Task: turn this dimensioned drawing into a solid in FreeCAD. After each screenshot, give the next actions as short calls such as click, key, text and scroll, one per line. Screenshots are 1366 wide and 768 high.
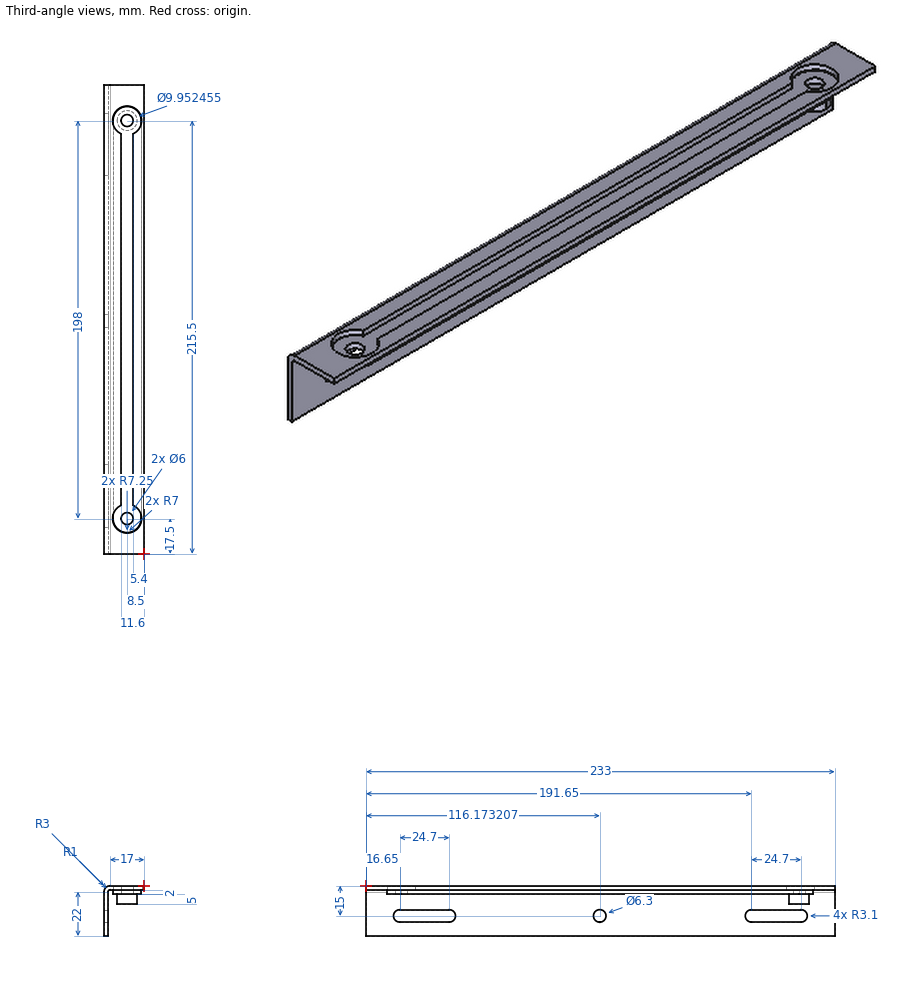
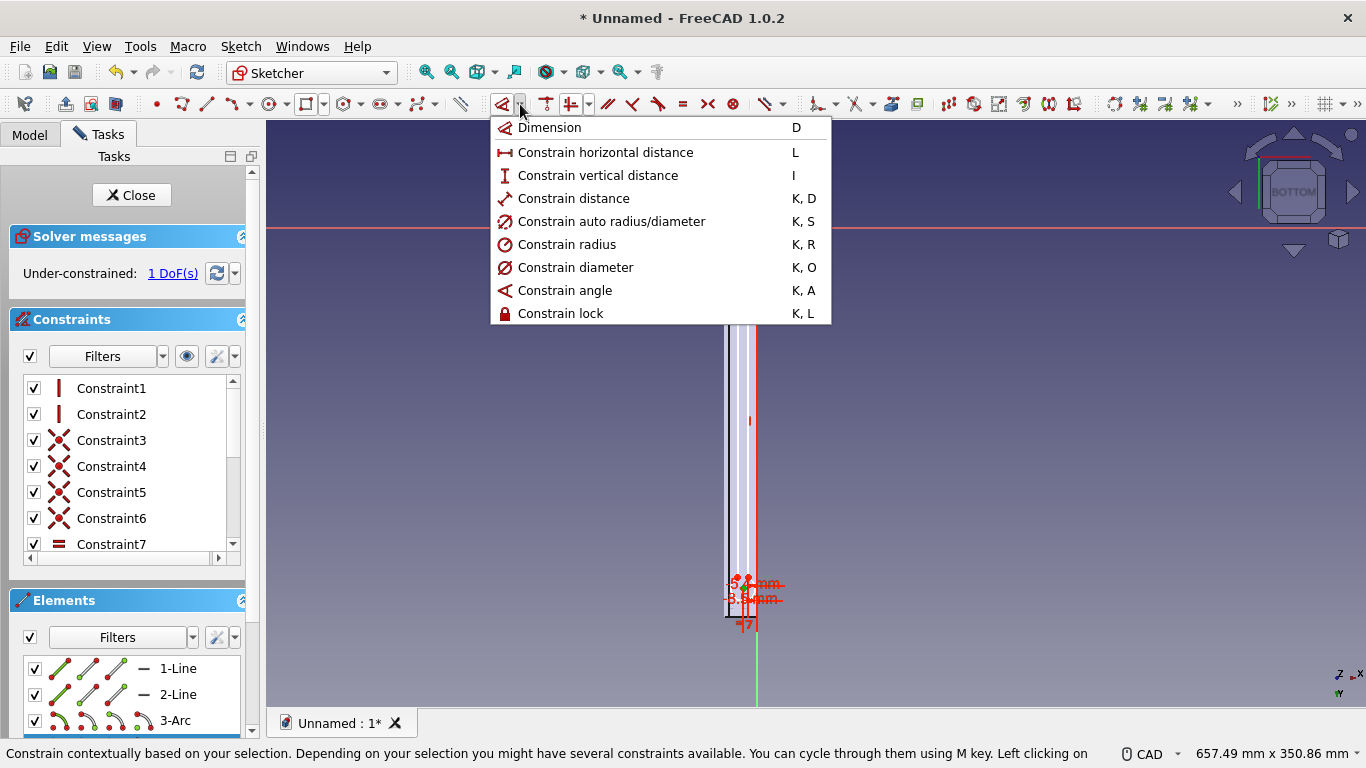
click(661, 176)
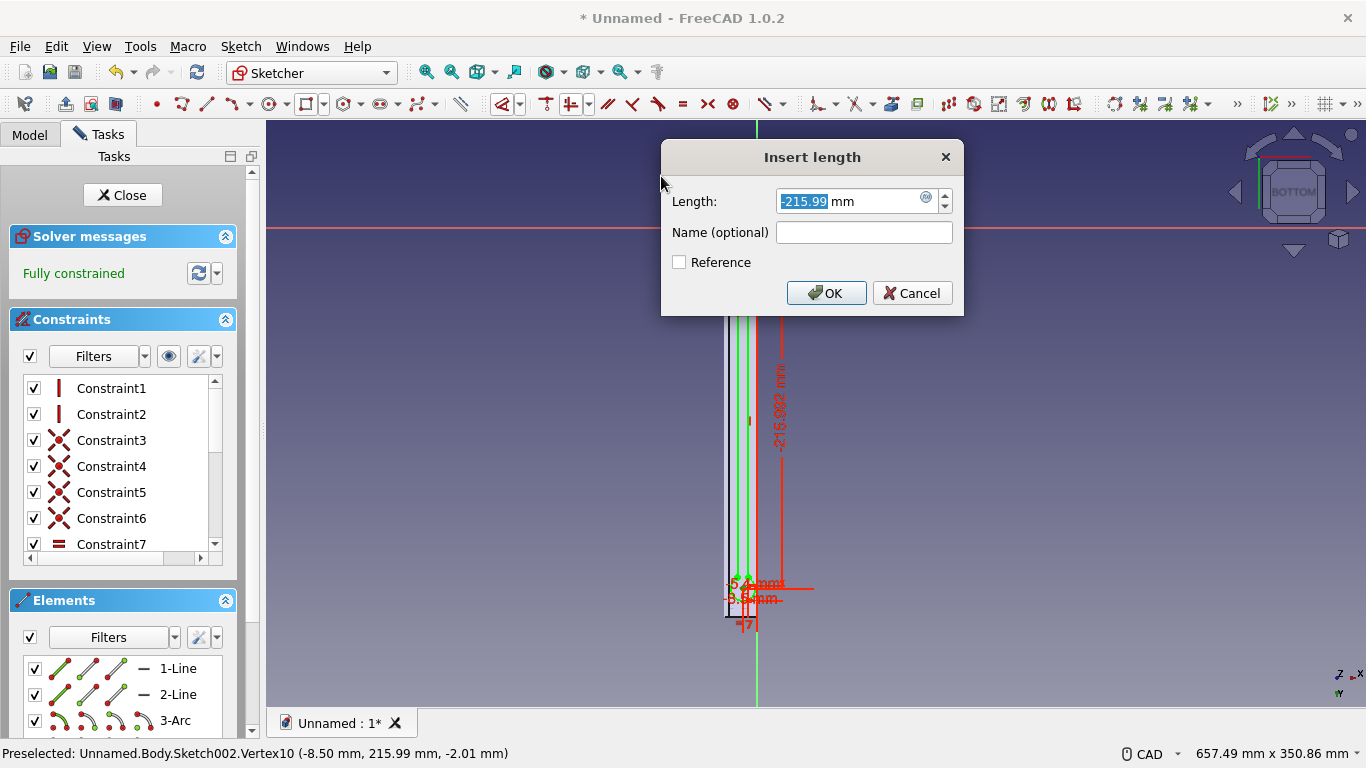
text(-215.5)
key(Return)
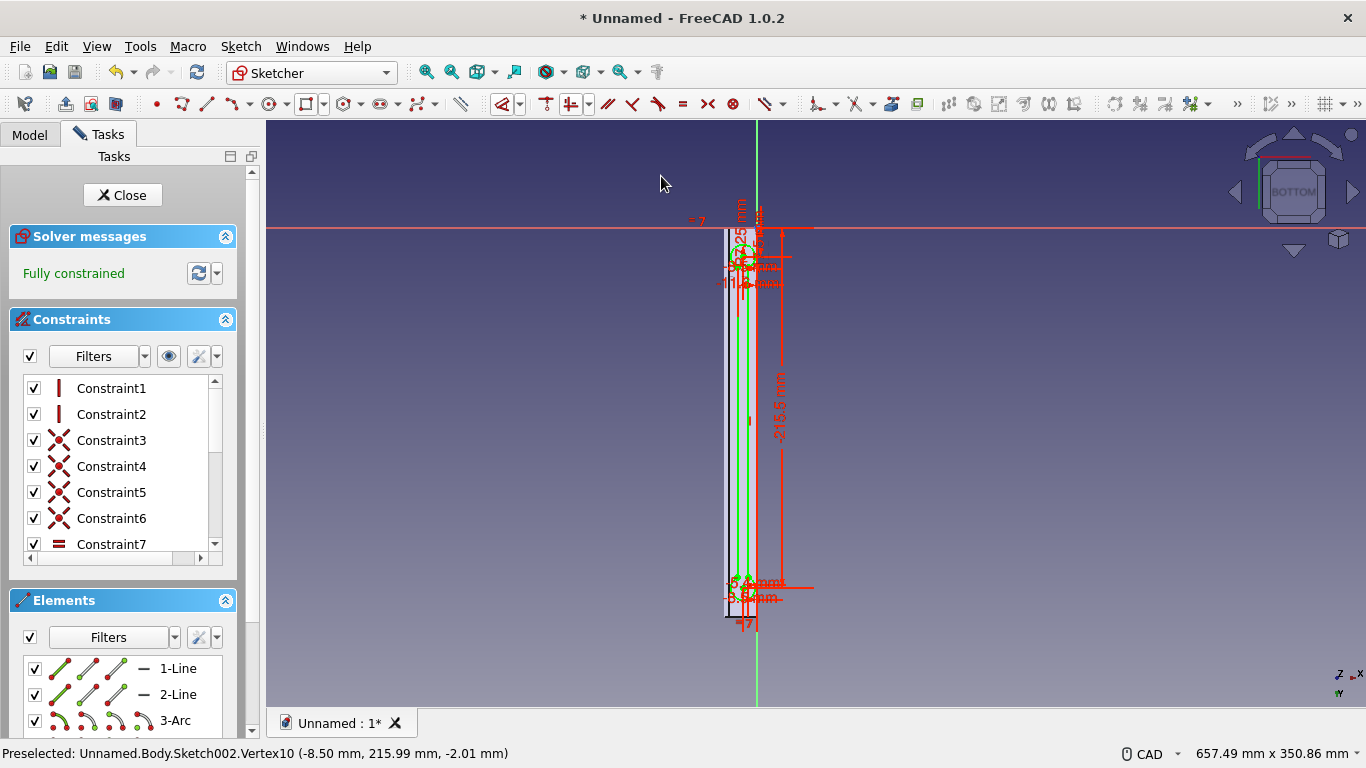
click(123, 195)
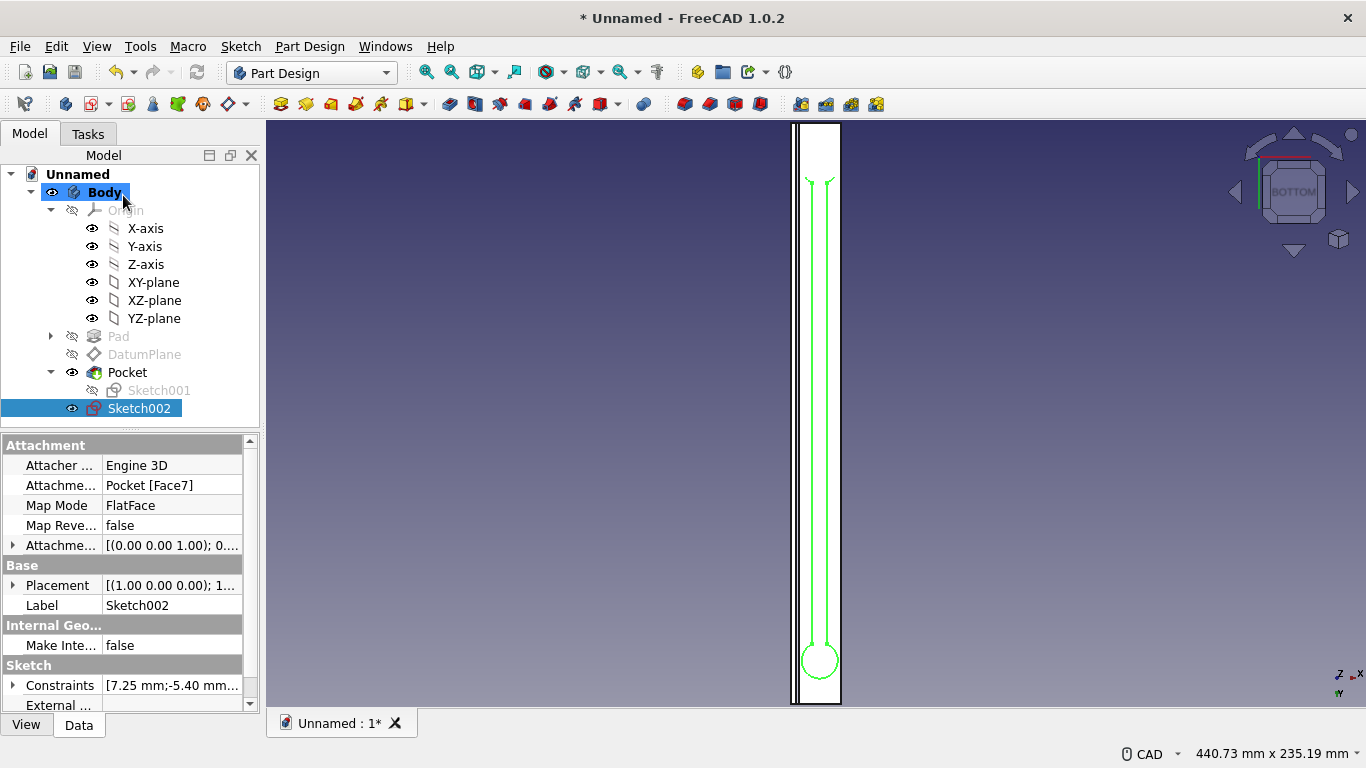
click(450, 104)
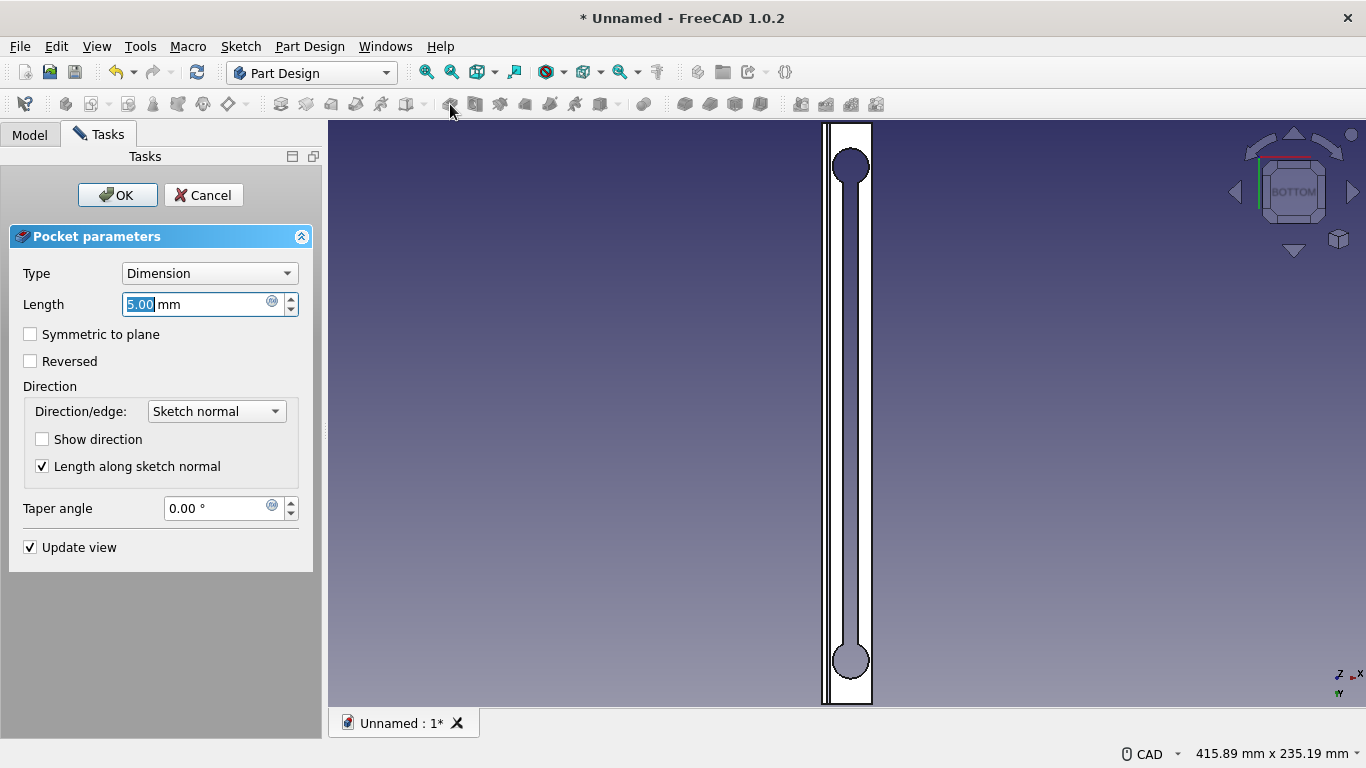
click(210, 274)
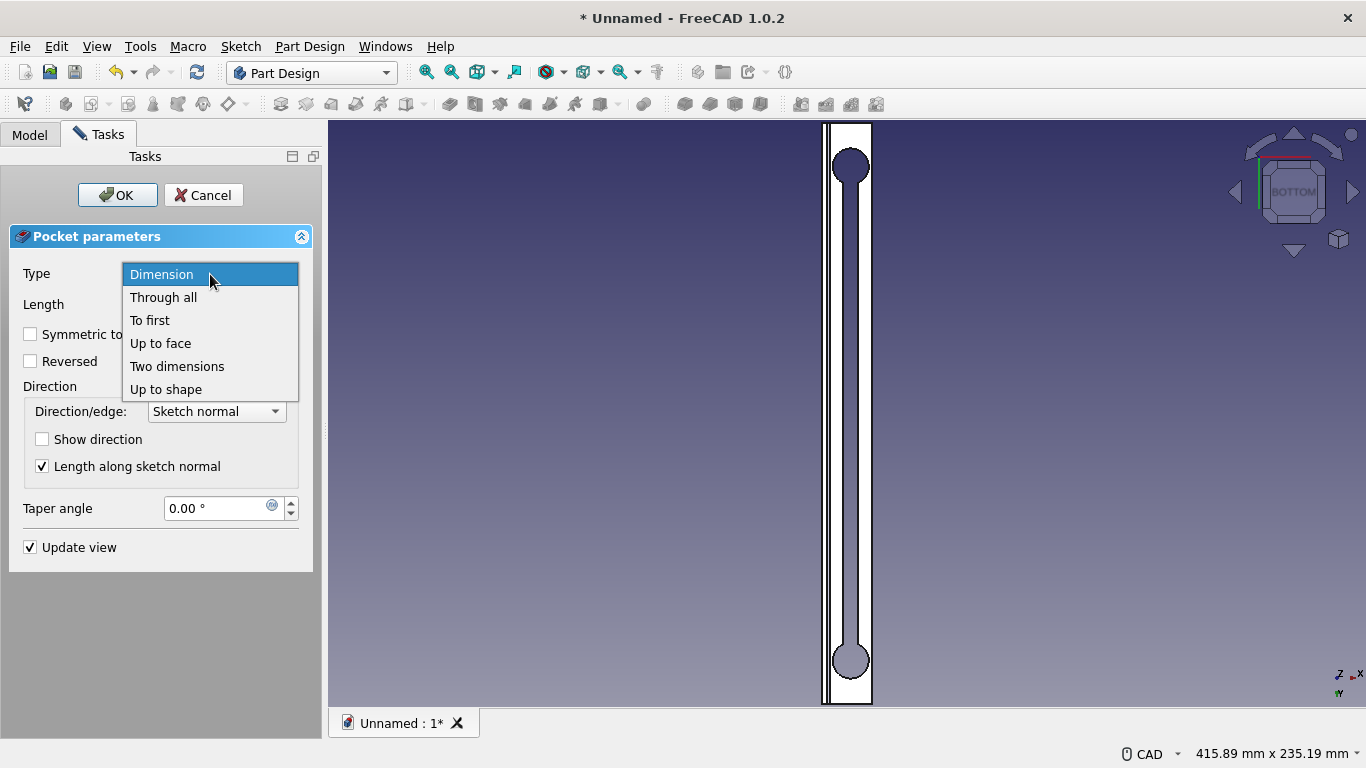
click(208, 298)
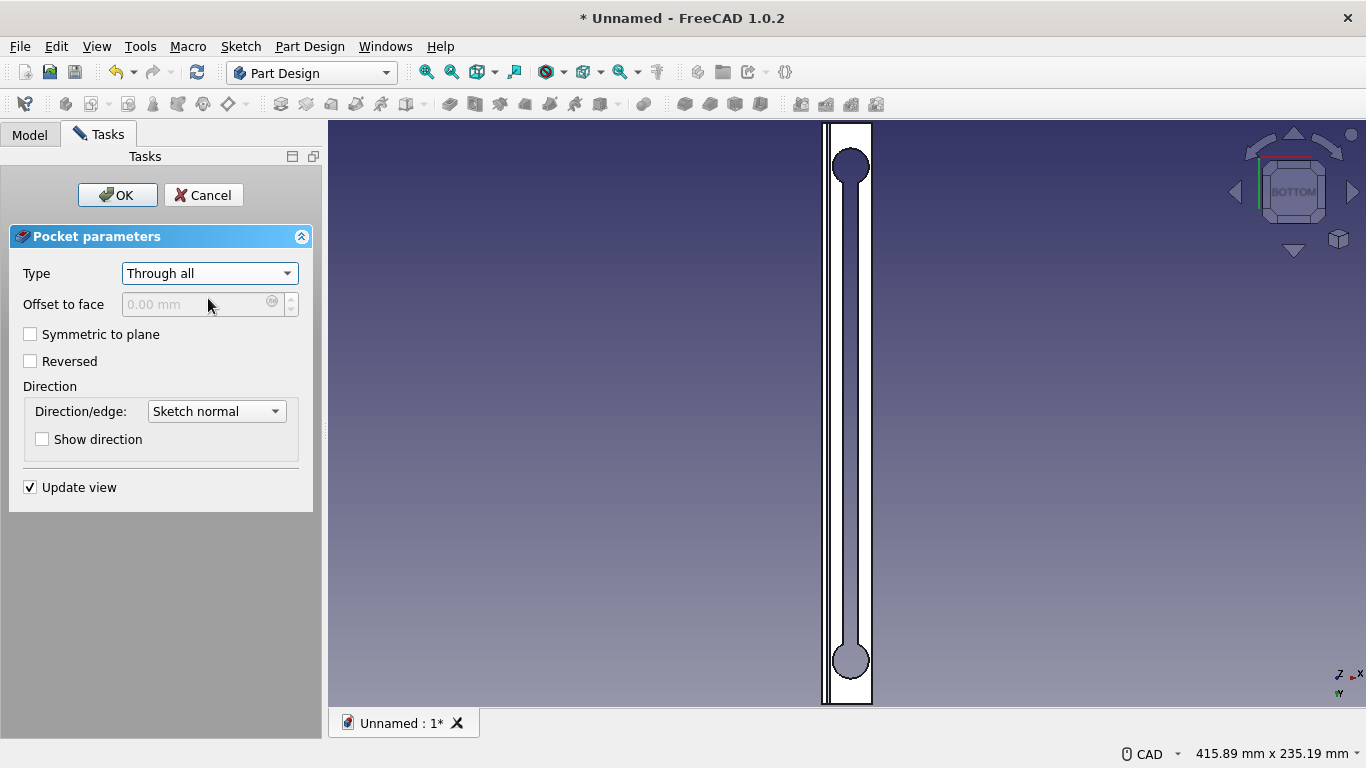
click(118, 195)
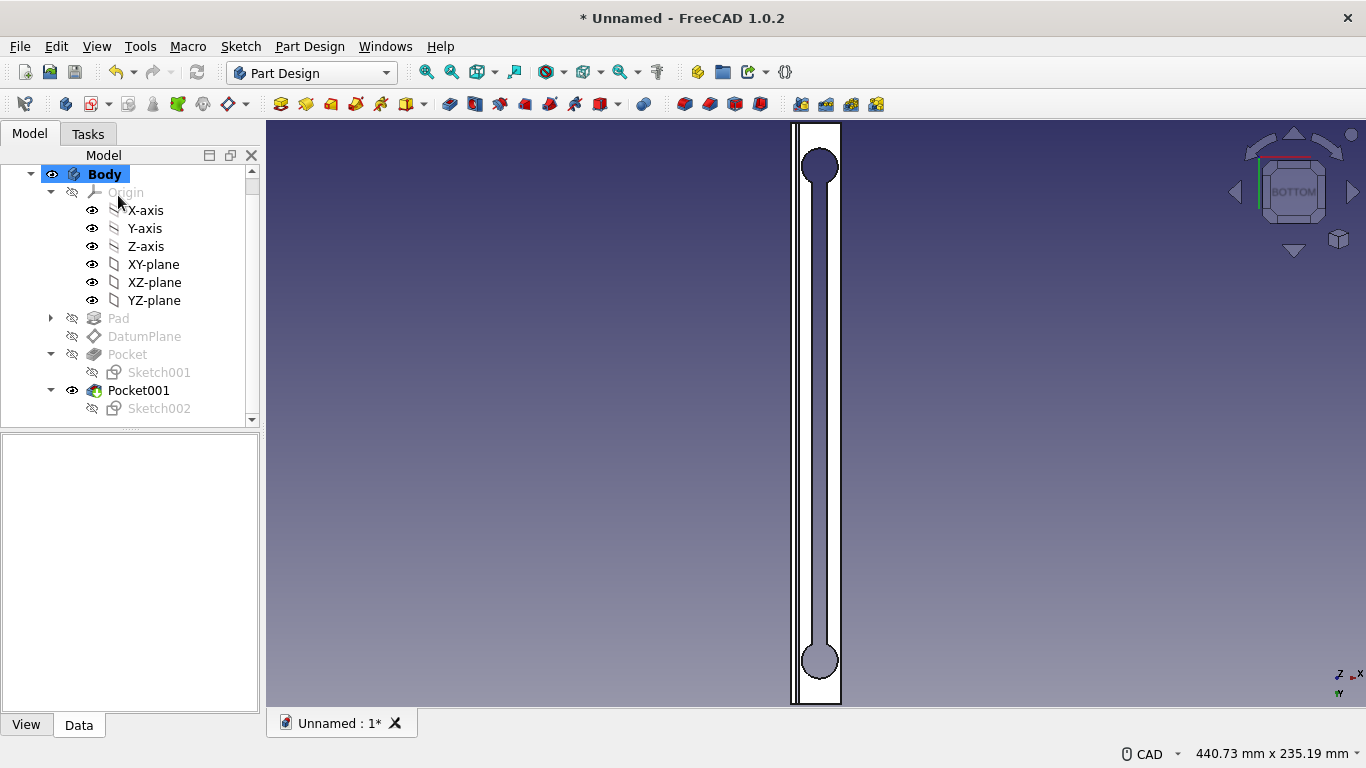
scroll(808, 579, up, 6)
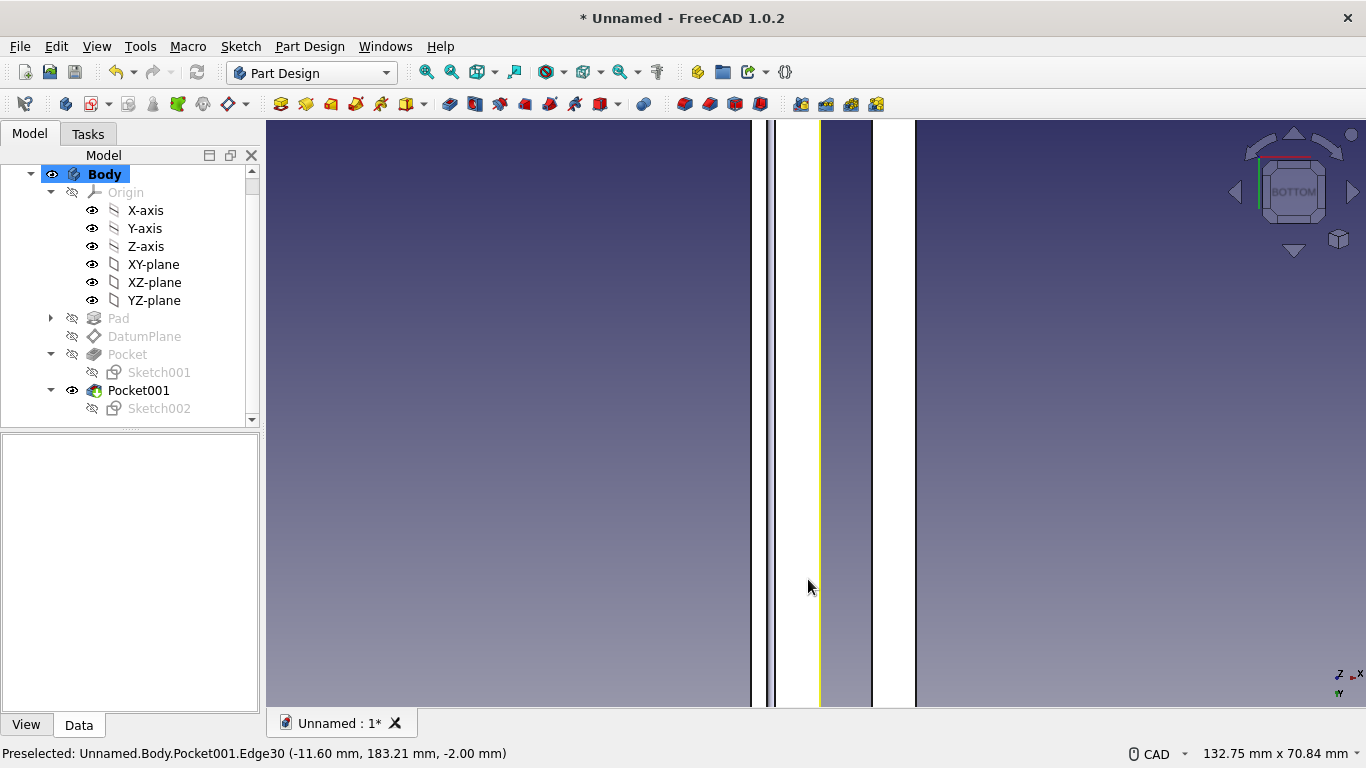
click(806, 578)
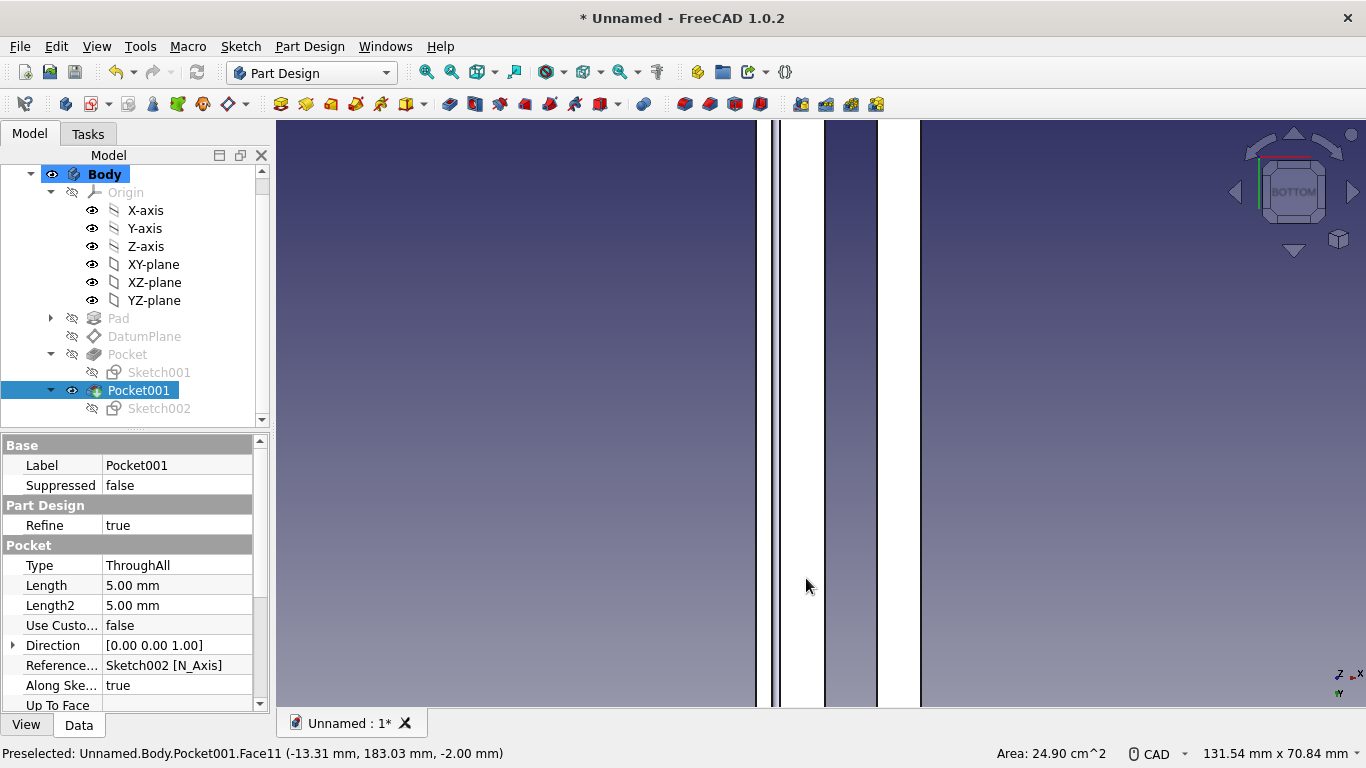
click(90, 104)